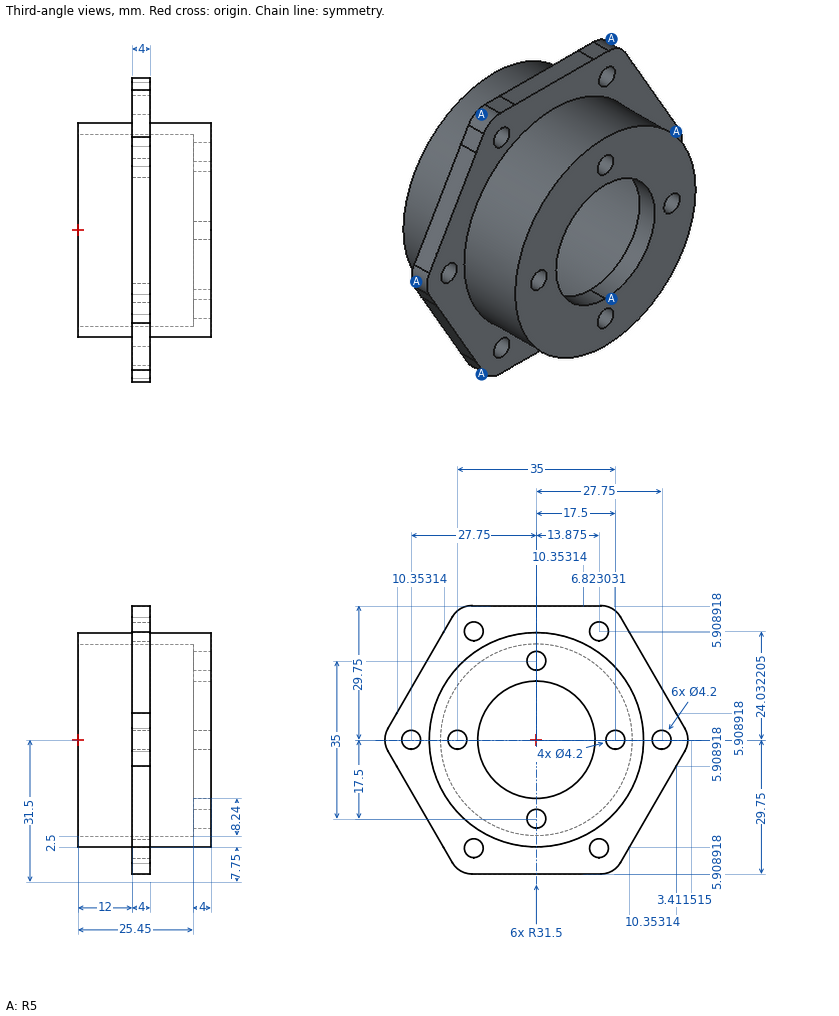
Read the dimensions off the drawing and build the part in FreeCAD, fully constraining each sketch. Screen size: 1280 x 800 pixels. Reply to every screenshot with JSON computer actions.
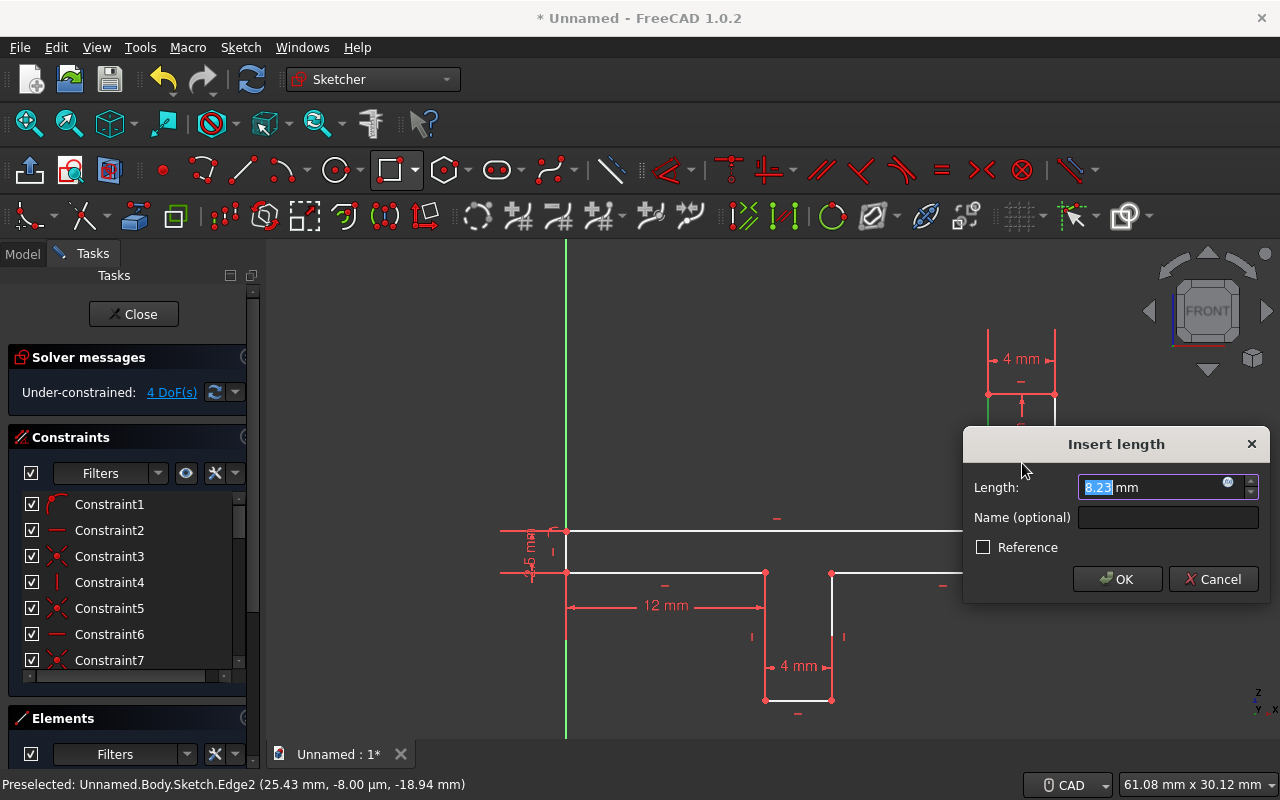
{"action": "type", "text": "8.24"}
{"action": "key", "text": "Return"}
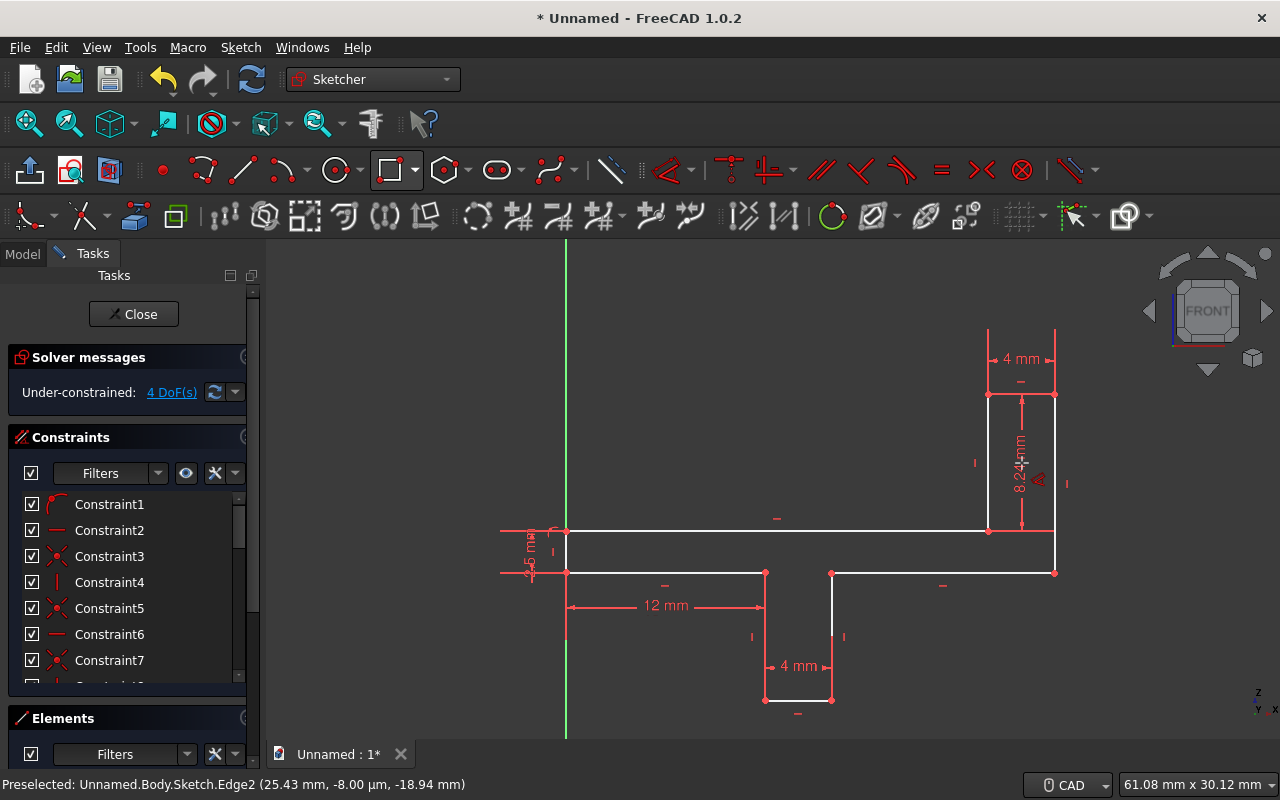
{"action": "left_click", "coordinate": [832, 611]}
{"action": "left_click", "coordinate": [866, 637]}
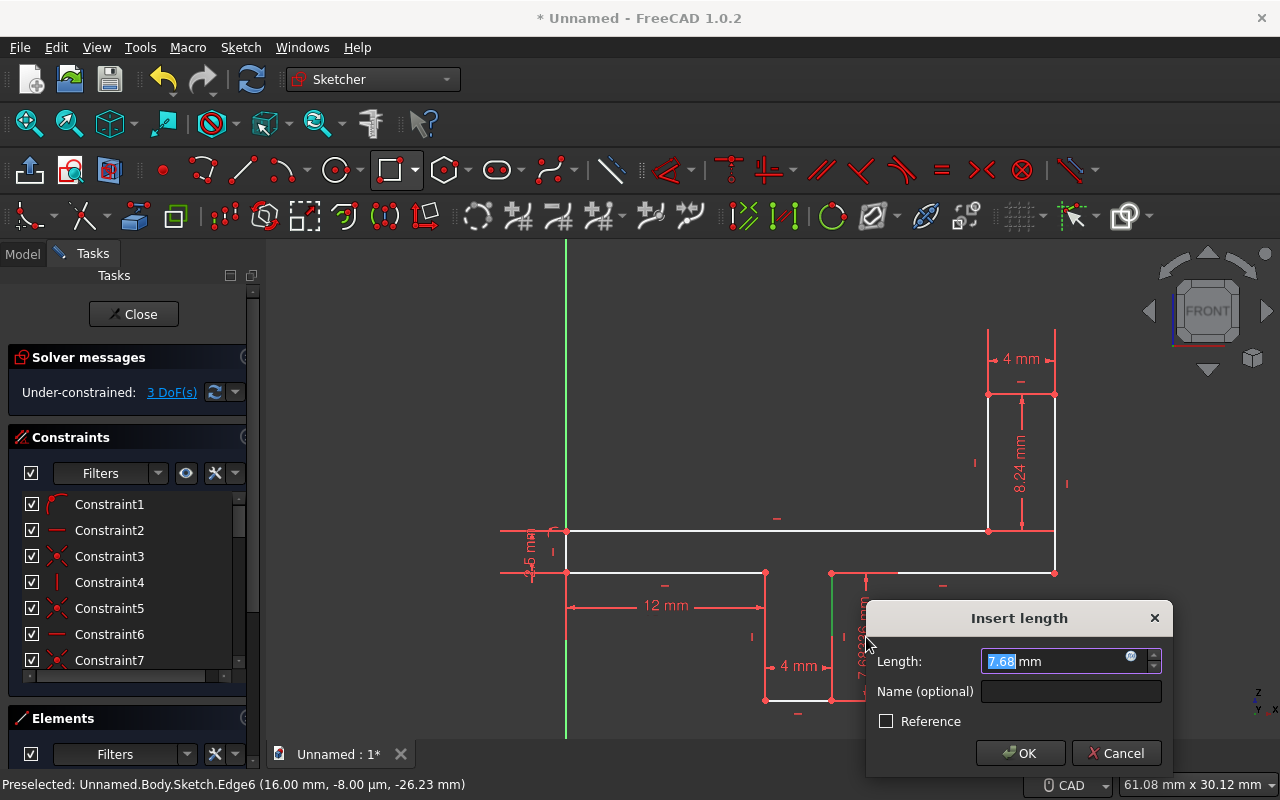
{"action": "type", "text": "7.75"}
{"action": "key", "text": "Return"}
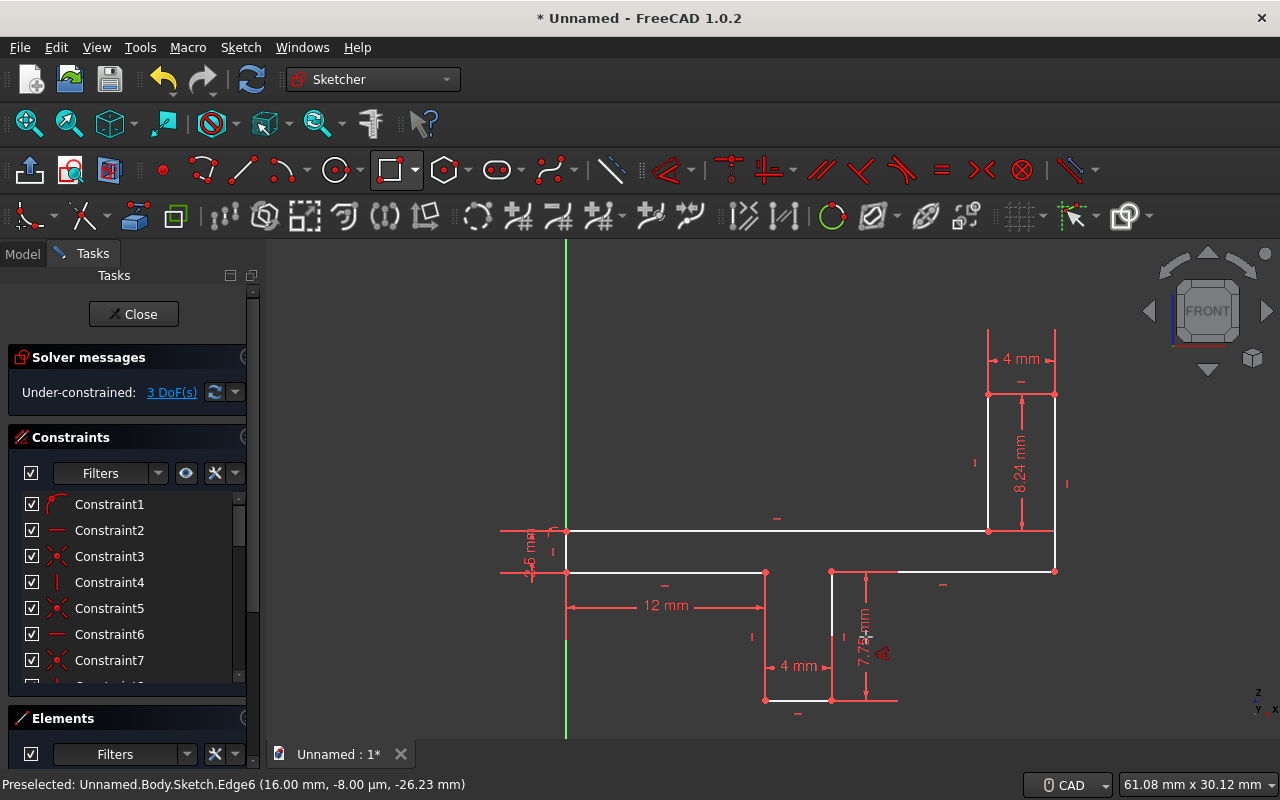
{"action": "left_click", "coordinate": [765, 662]}
{"action": "left_click", "coordinate": [731, 637]}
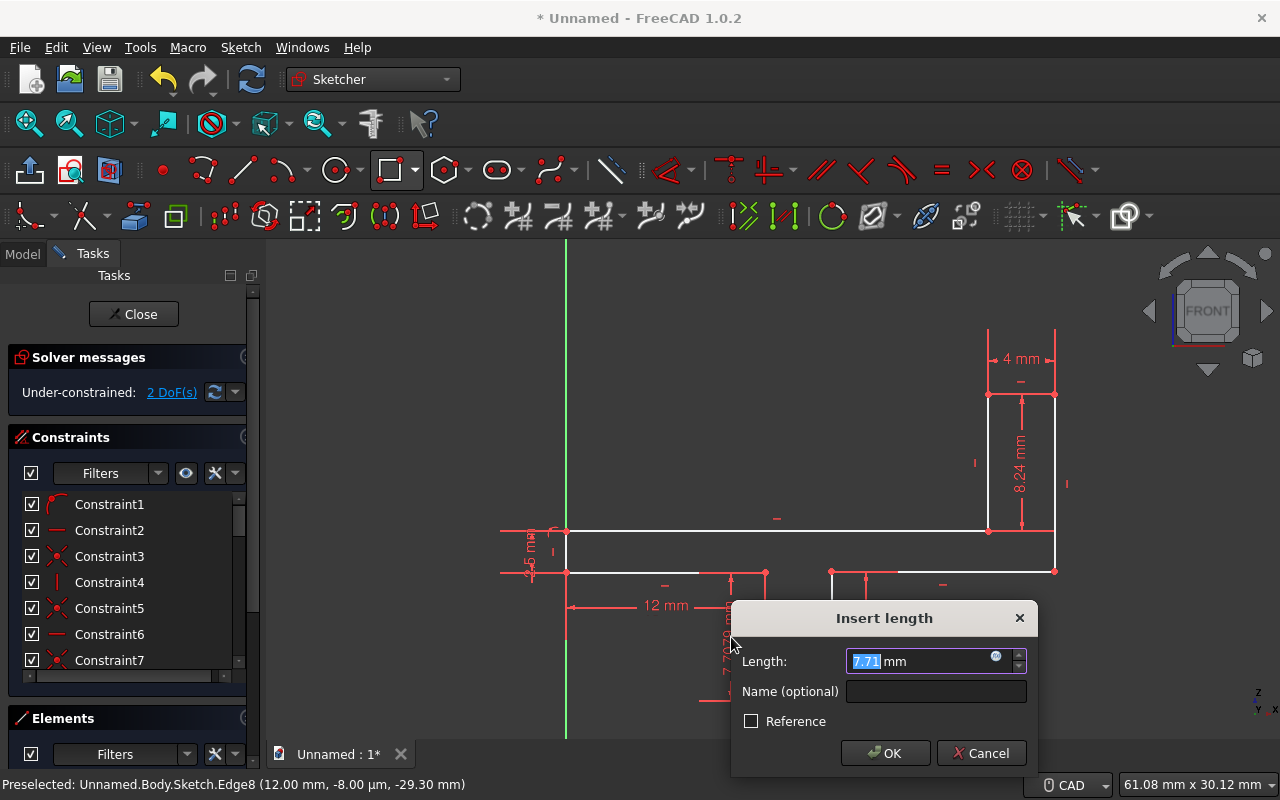
{"action": "type", "text": "7.75"}
{"action": "key", "text": "Return"}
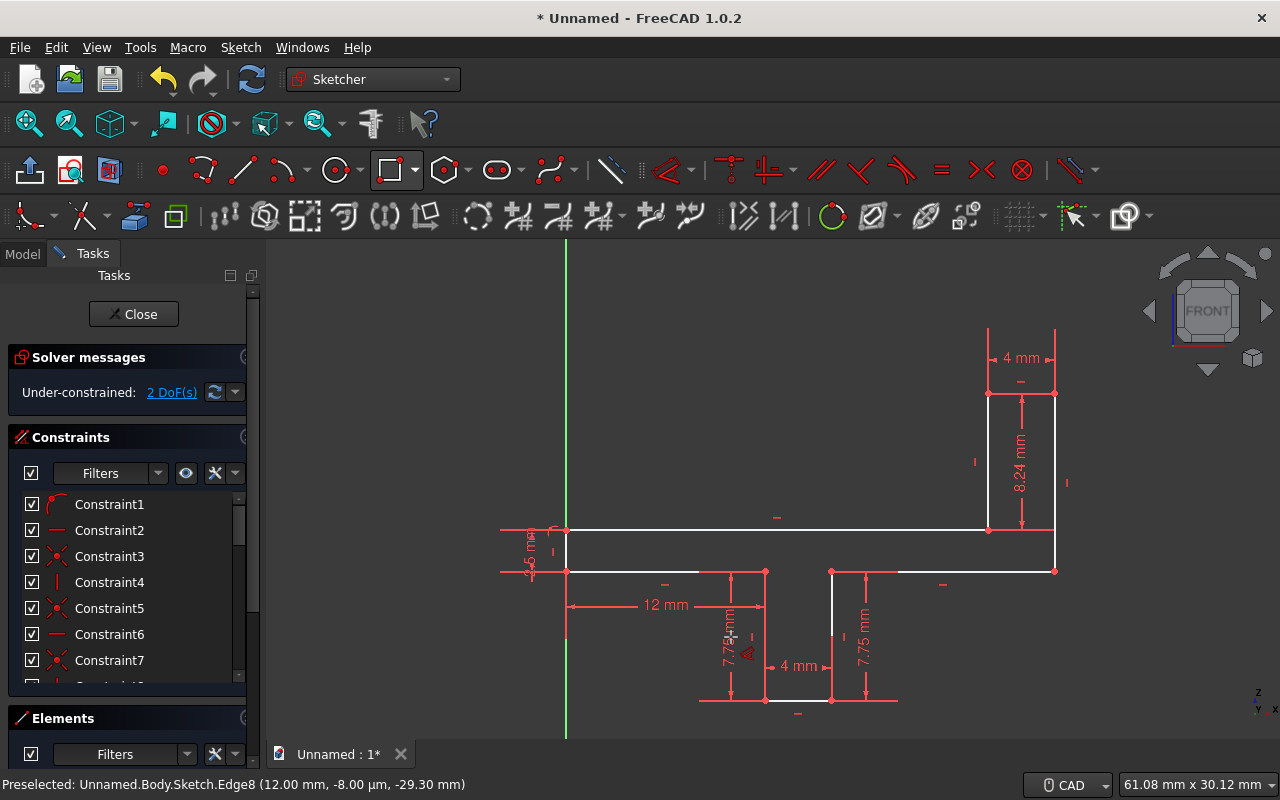
{"action": "left_click", "coordinate": [693, 530]}
{"action": "left_click", "coordinate": [777, 564]}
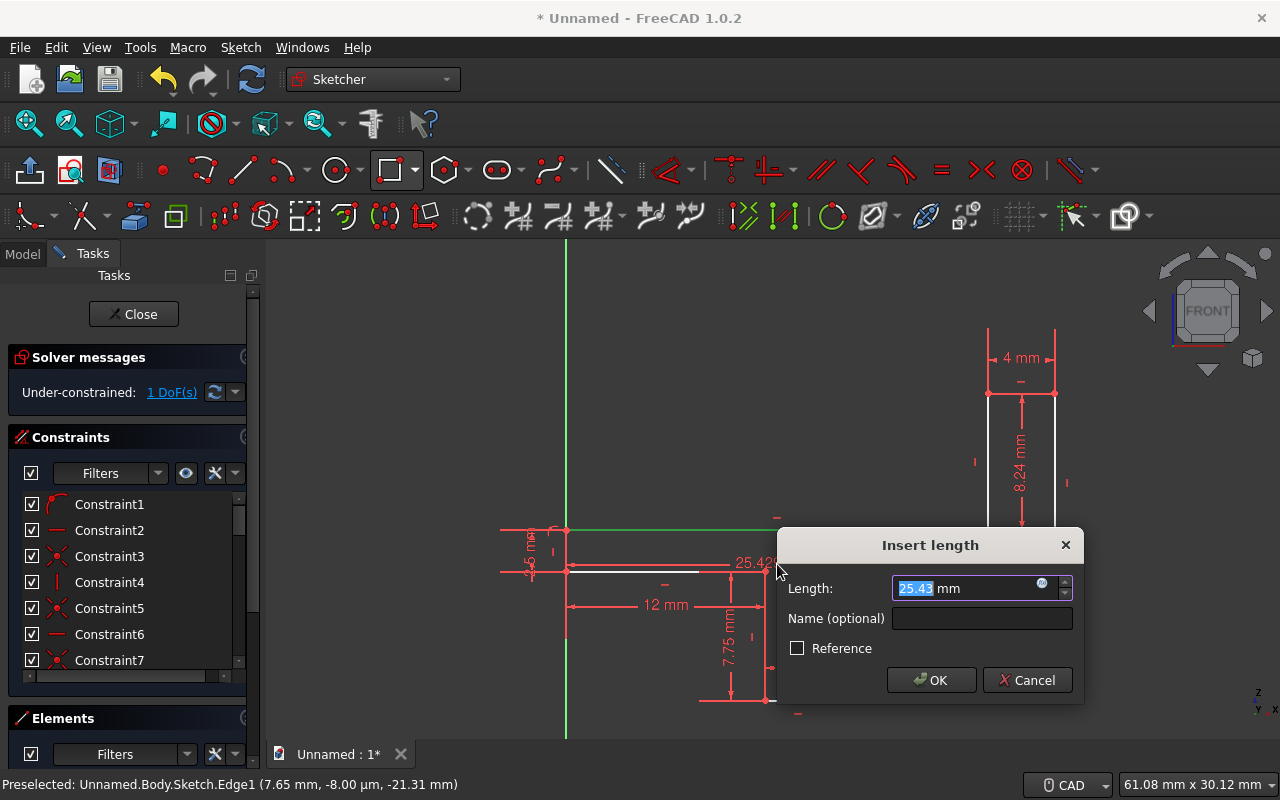
{"action": "type", "text": "25.45"}
{"action": "key", "text": "Return"}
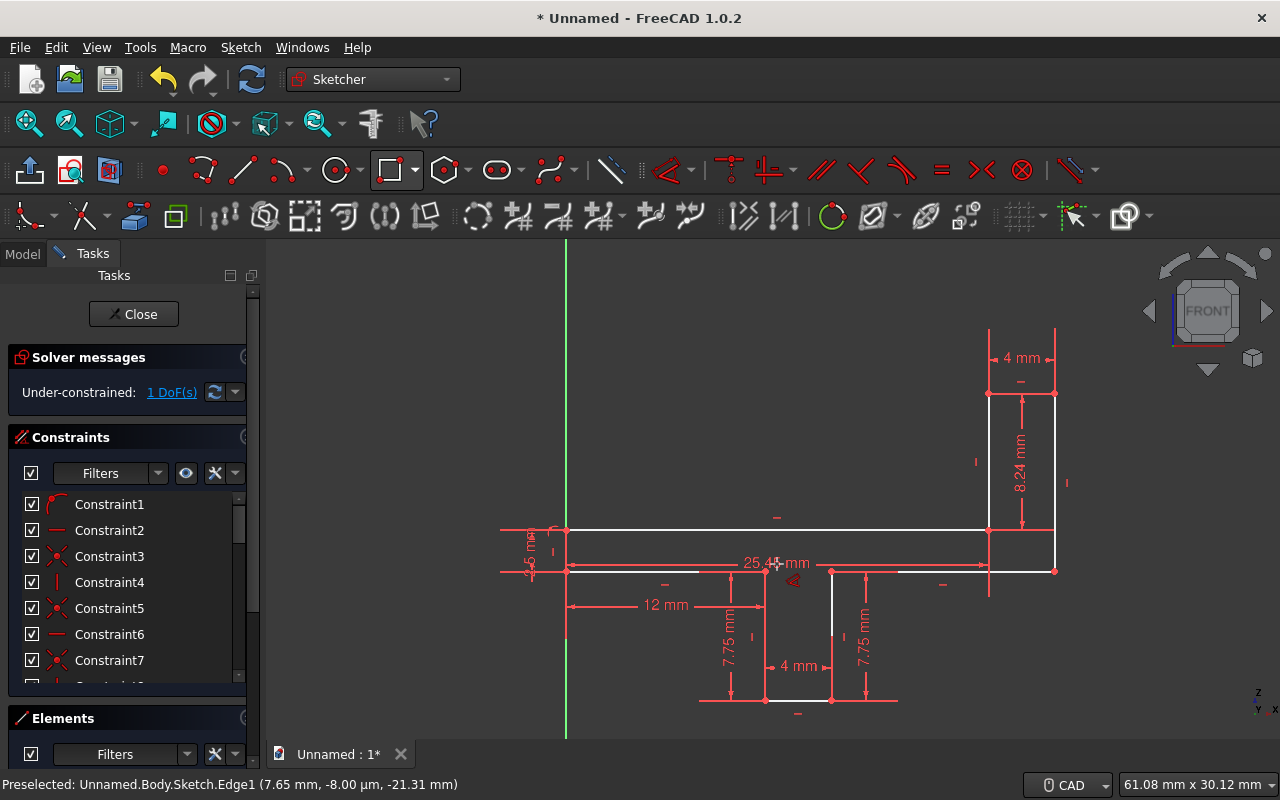
{"action": "left_click", "coordinate": [832, 701]}
{"action": "left_click", "coordinate": [532, 484]}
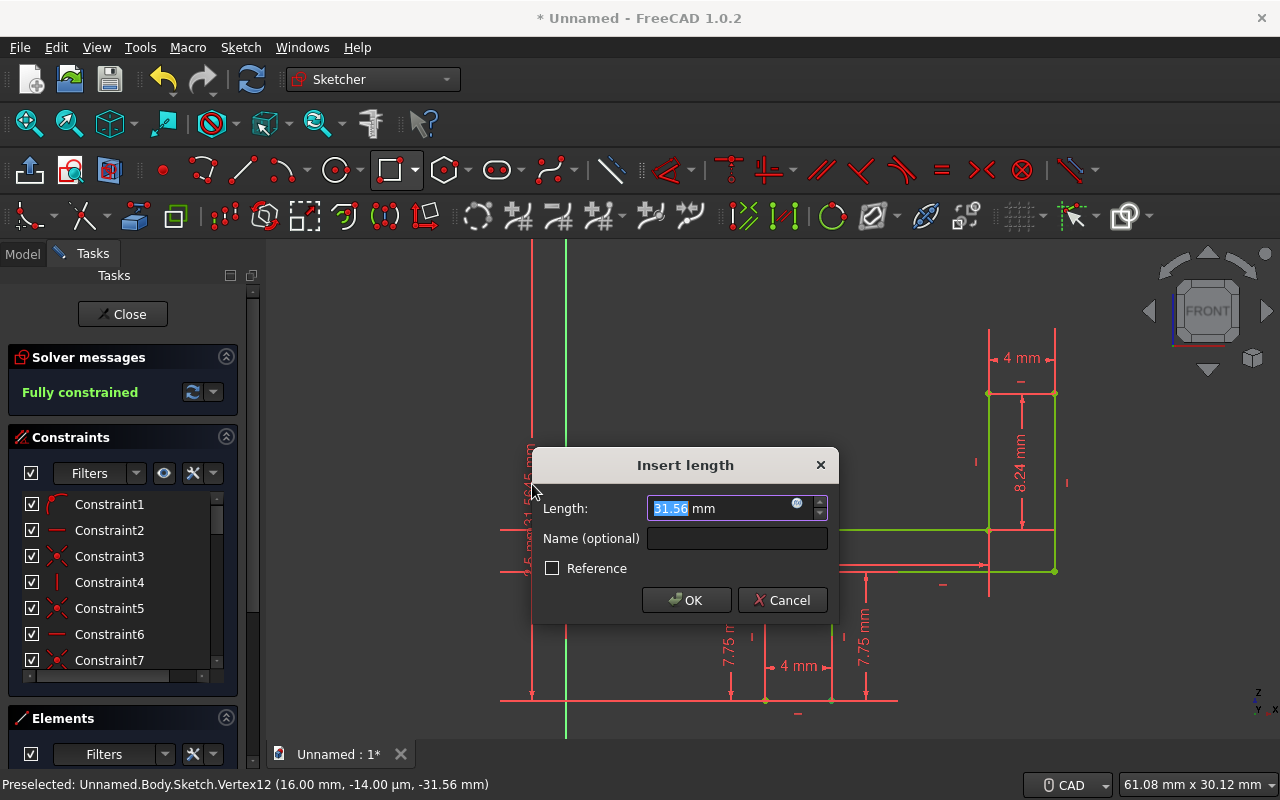
{"action": "type", "text": "31.5"}
{"action": "key", "text": "Return"}
{"action": "key", "text": "Escape"}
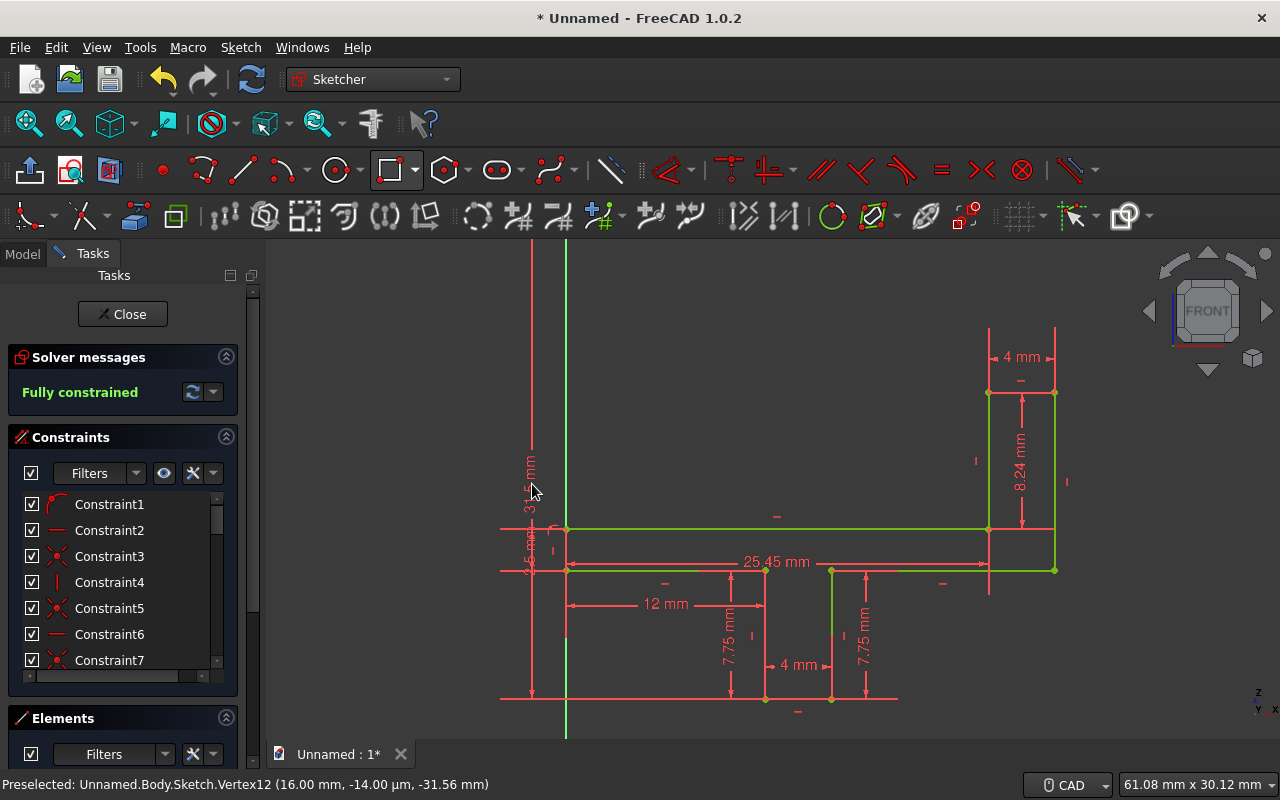
{"action": "left_click", "coordinate": [123, 314]}